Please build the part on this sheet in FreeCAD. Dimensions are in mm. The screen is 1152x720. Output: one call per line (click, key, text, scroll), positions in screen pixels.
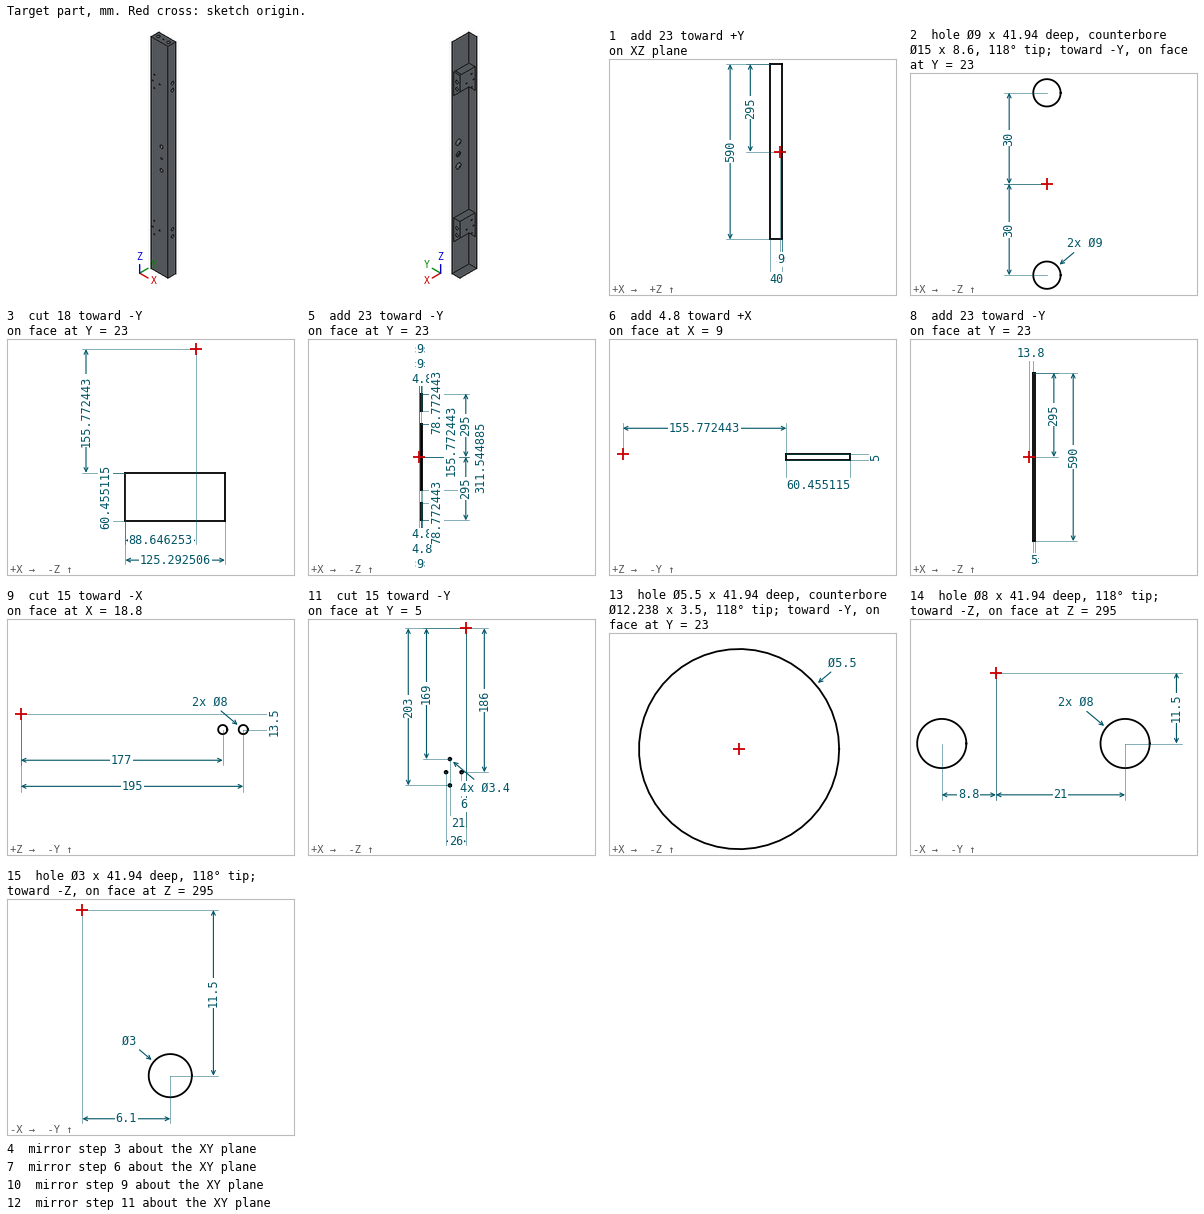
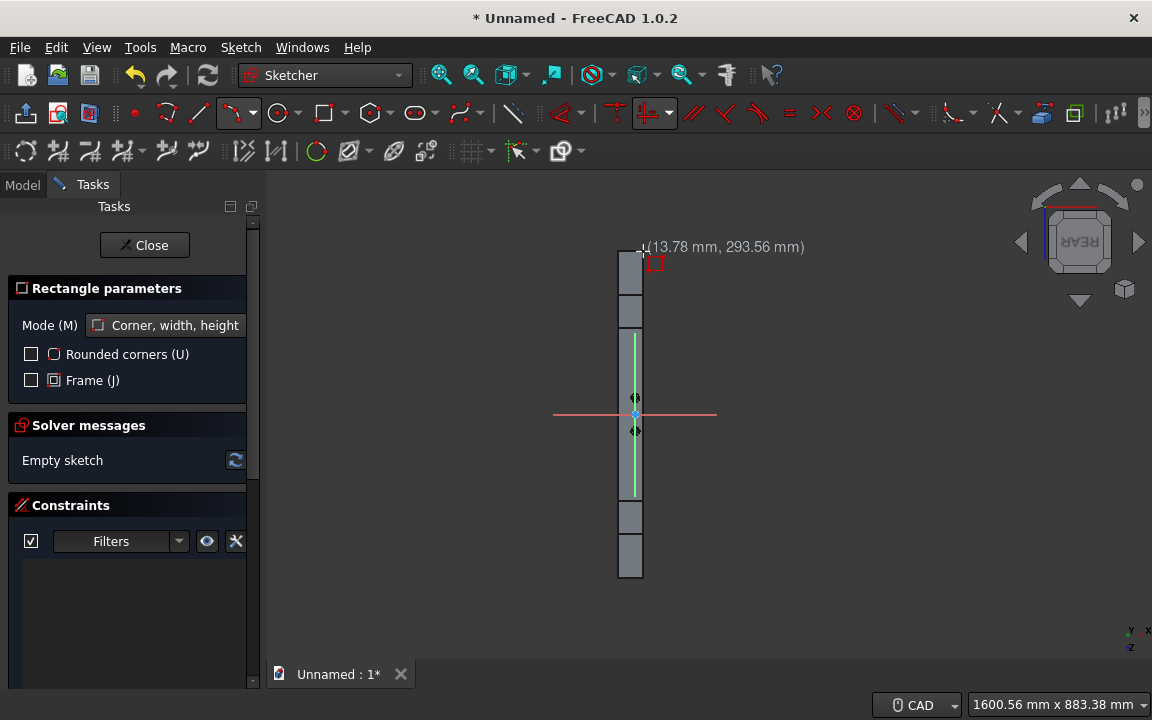
scroll(643, 251, up, 4)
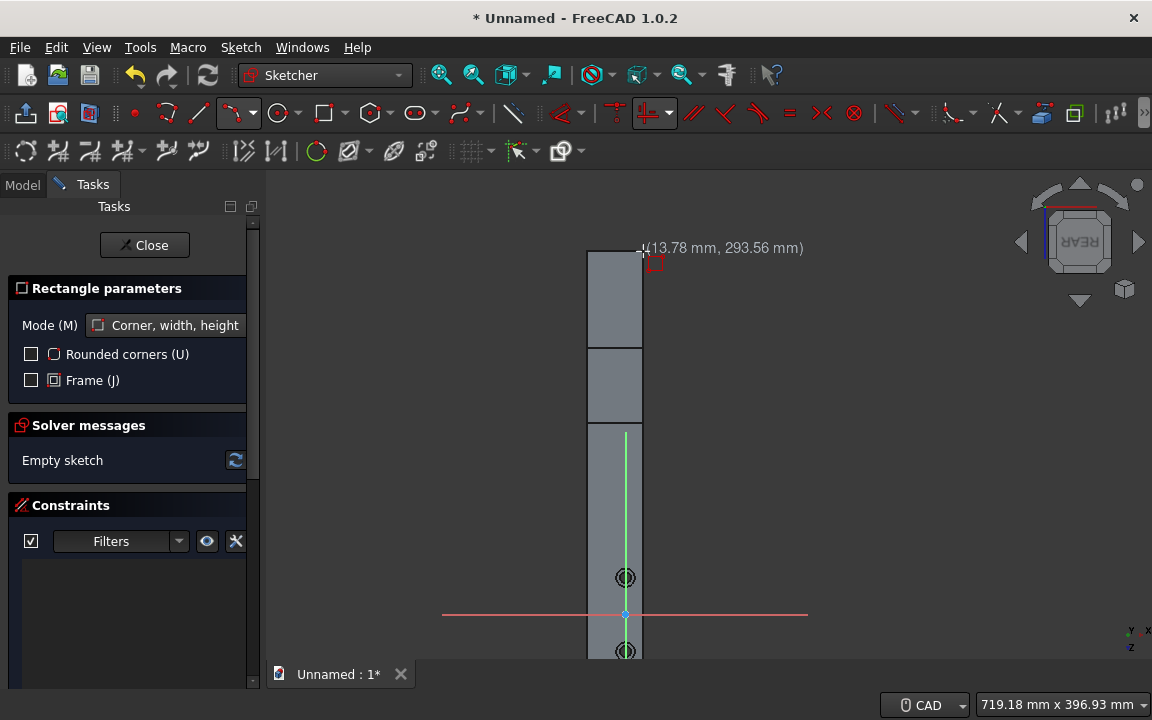
click(643, 251)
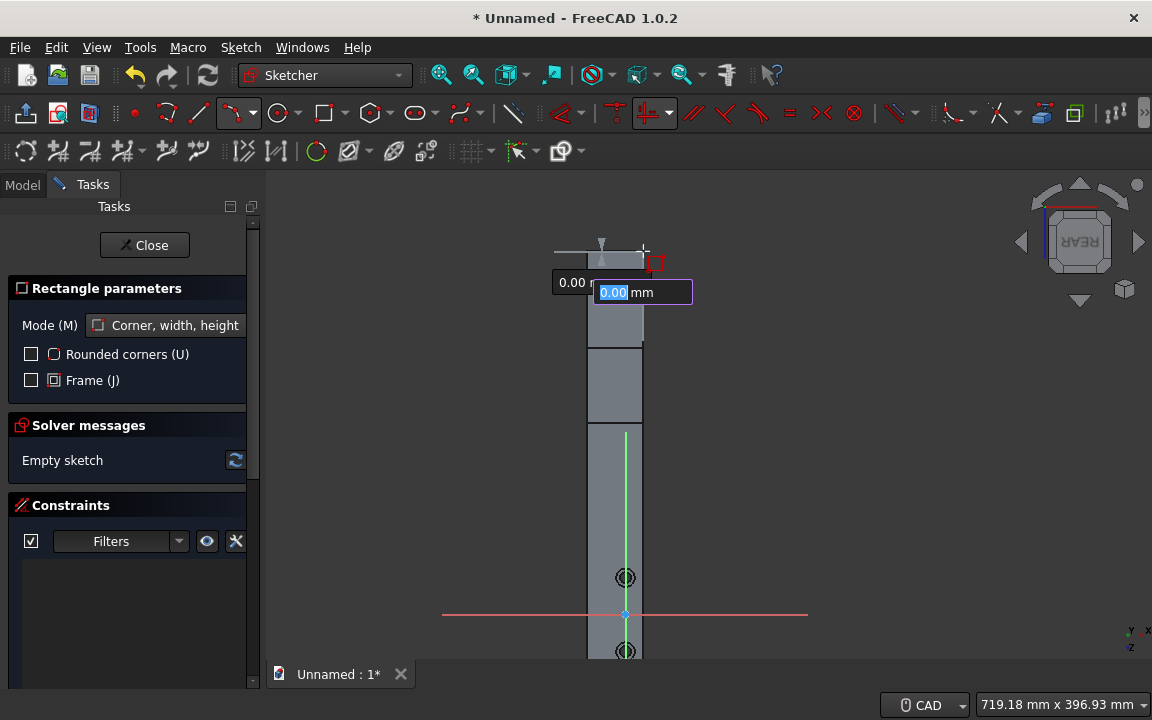
scroll(643, 251, down, 4)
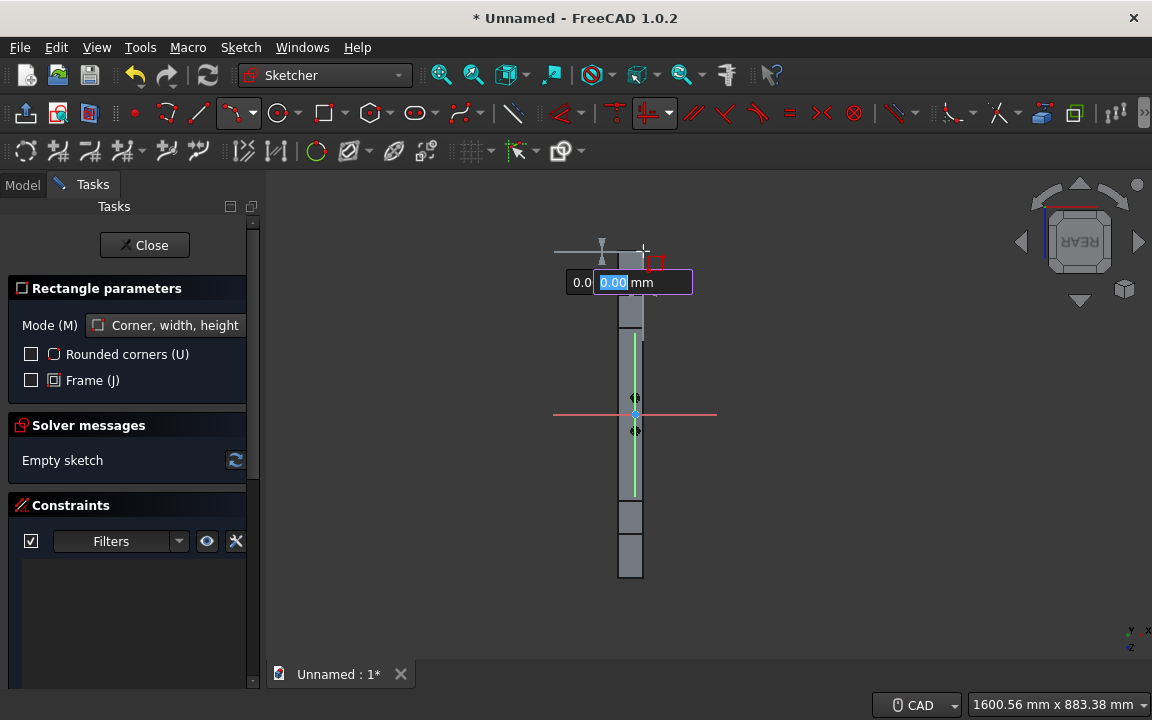
scroll(646, 578, up, 3)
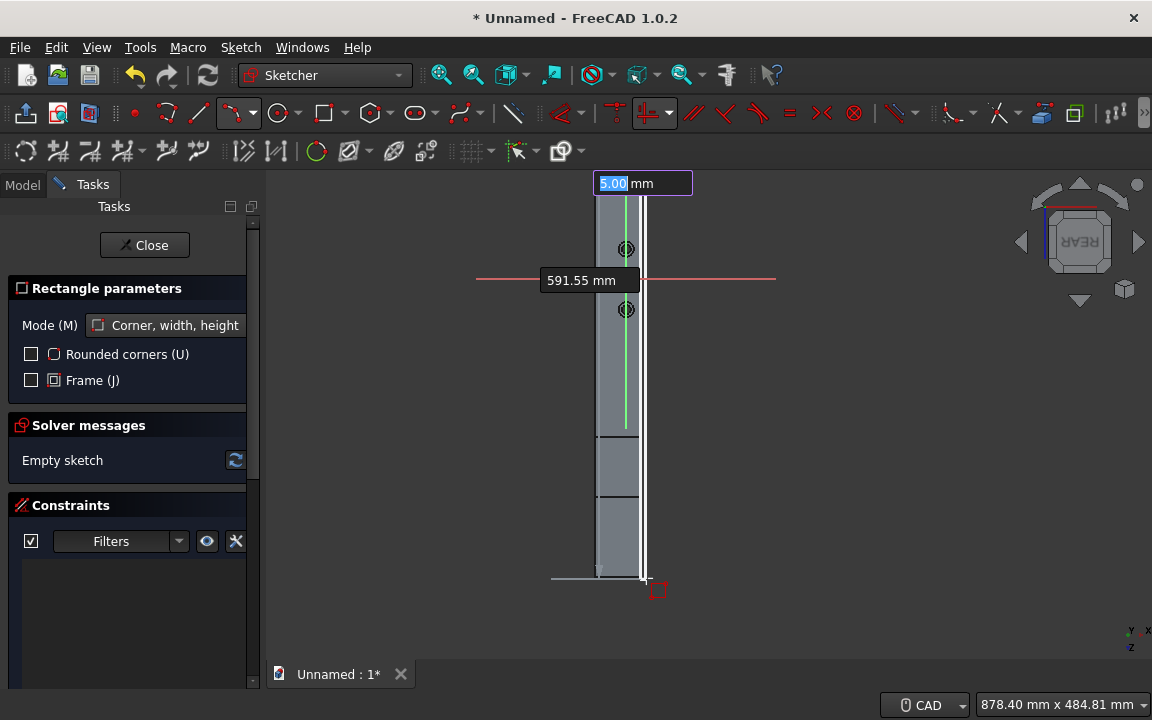
click(645, 577)
key(Escape)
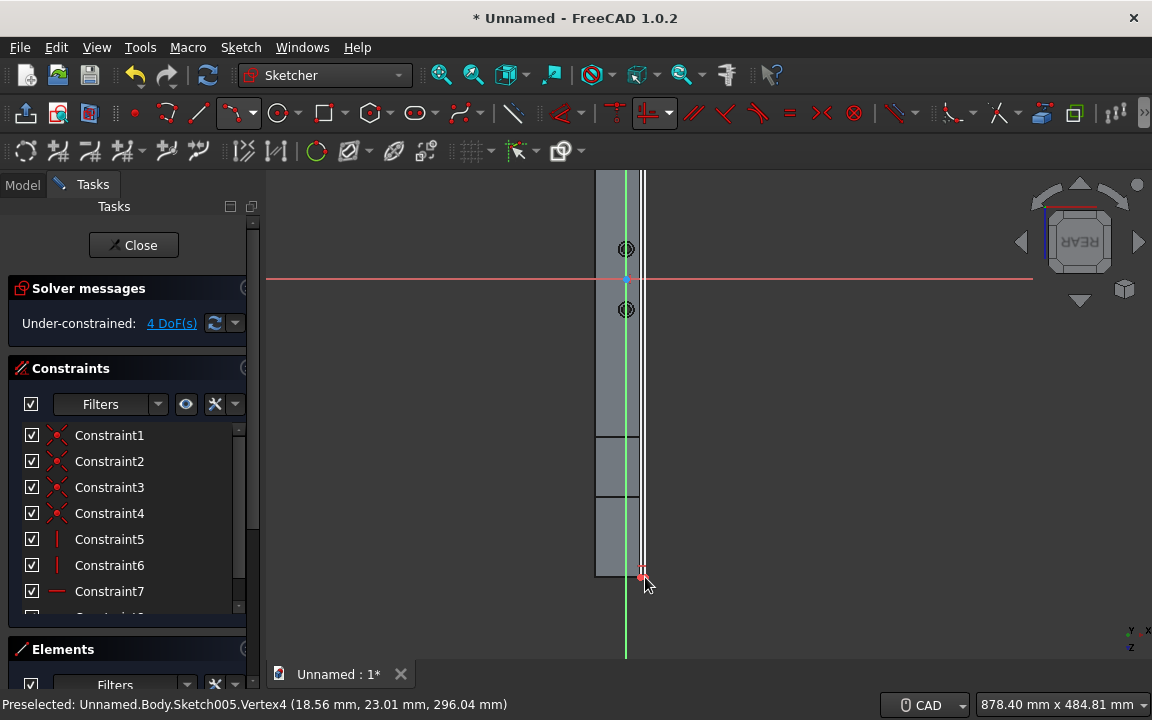
click(560, 114)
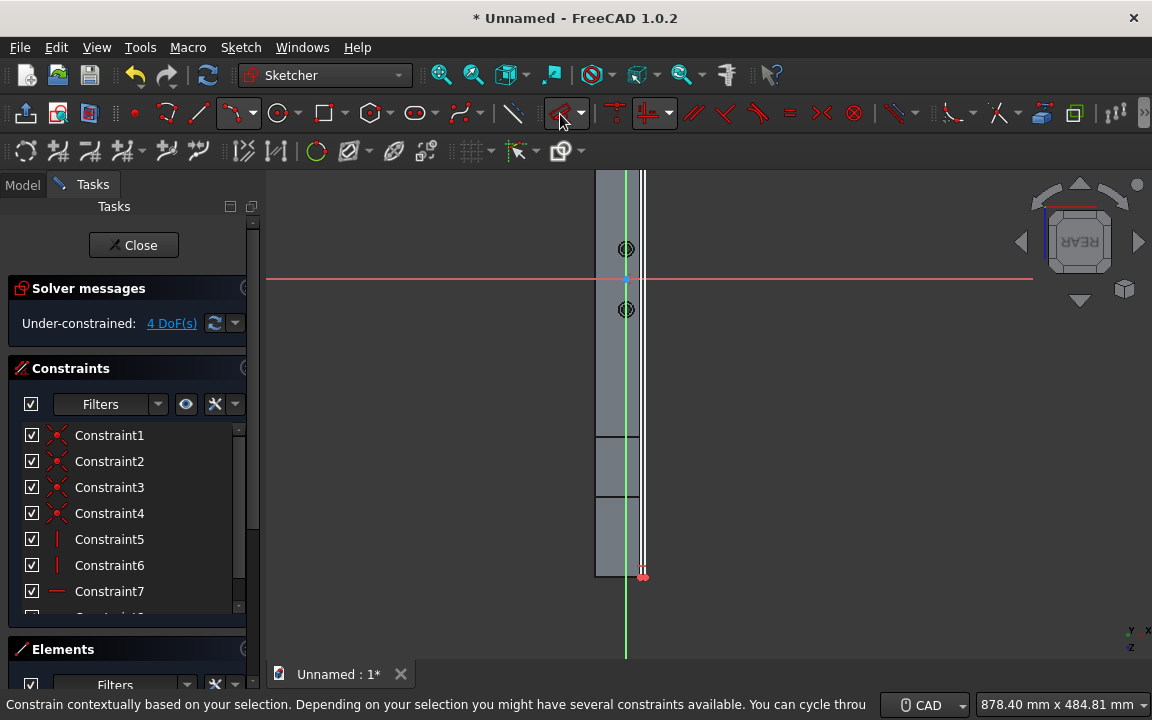
scroll(643, 578, up, 11)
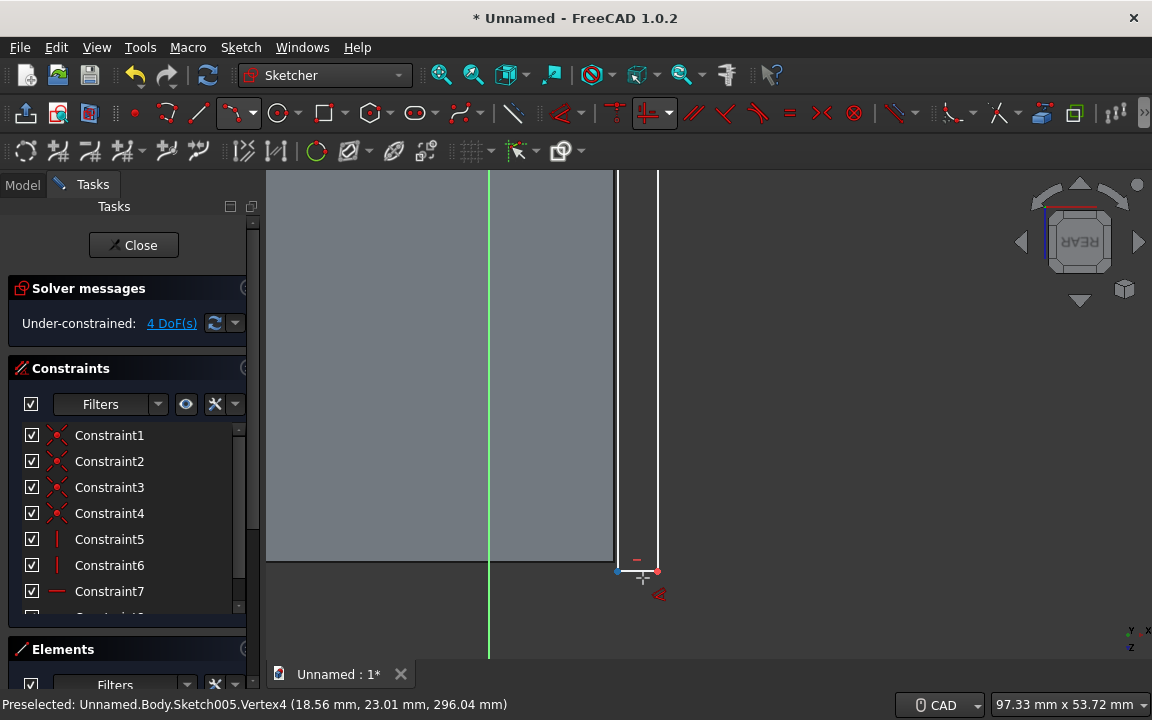
click(638, 571)
click(638, 605)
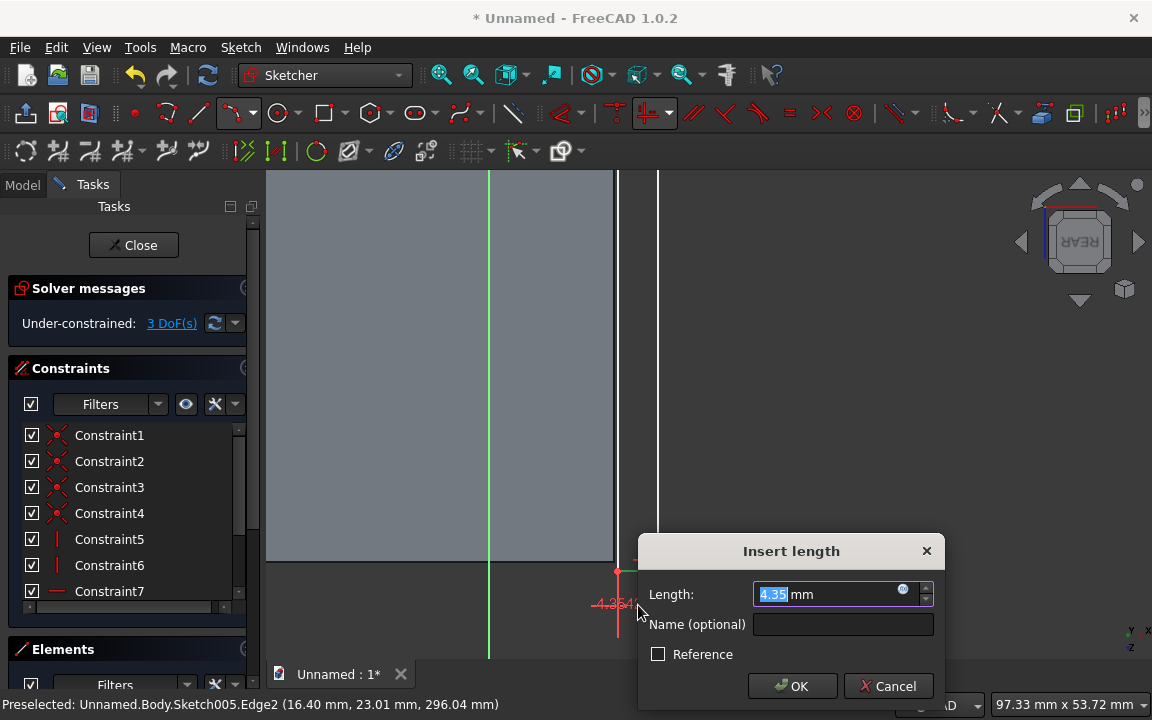
text(5)
key(Return)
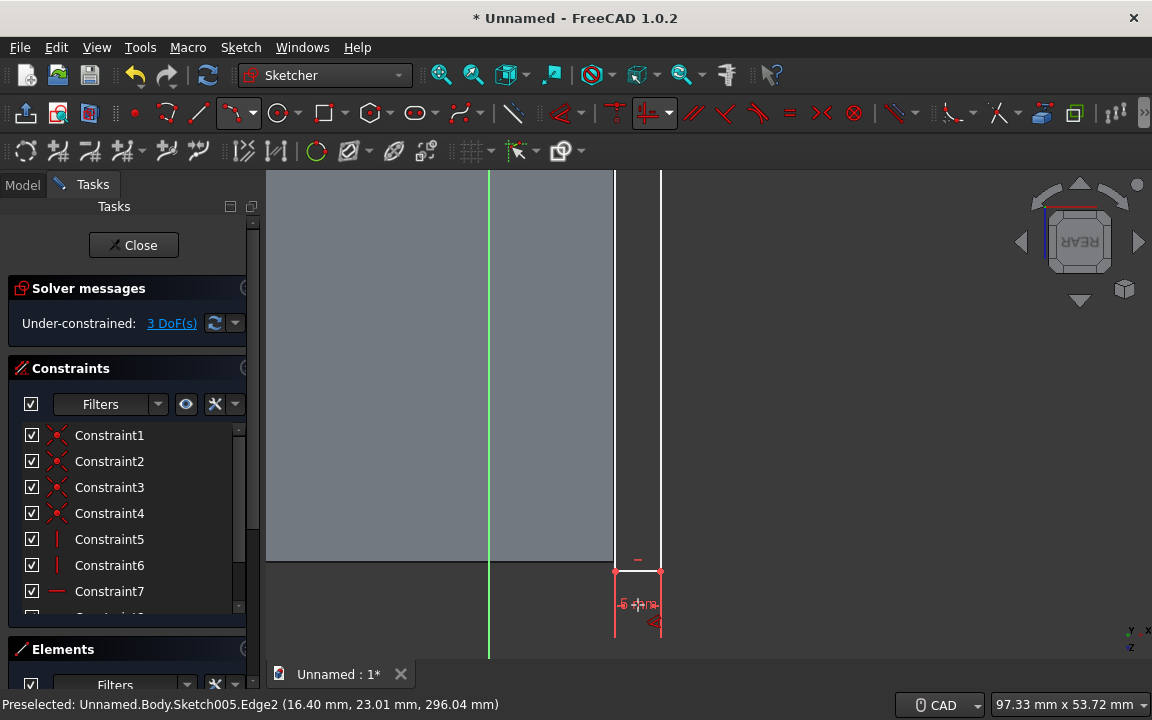
scroll(645, 579, down, 14)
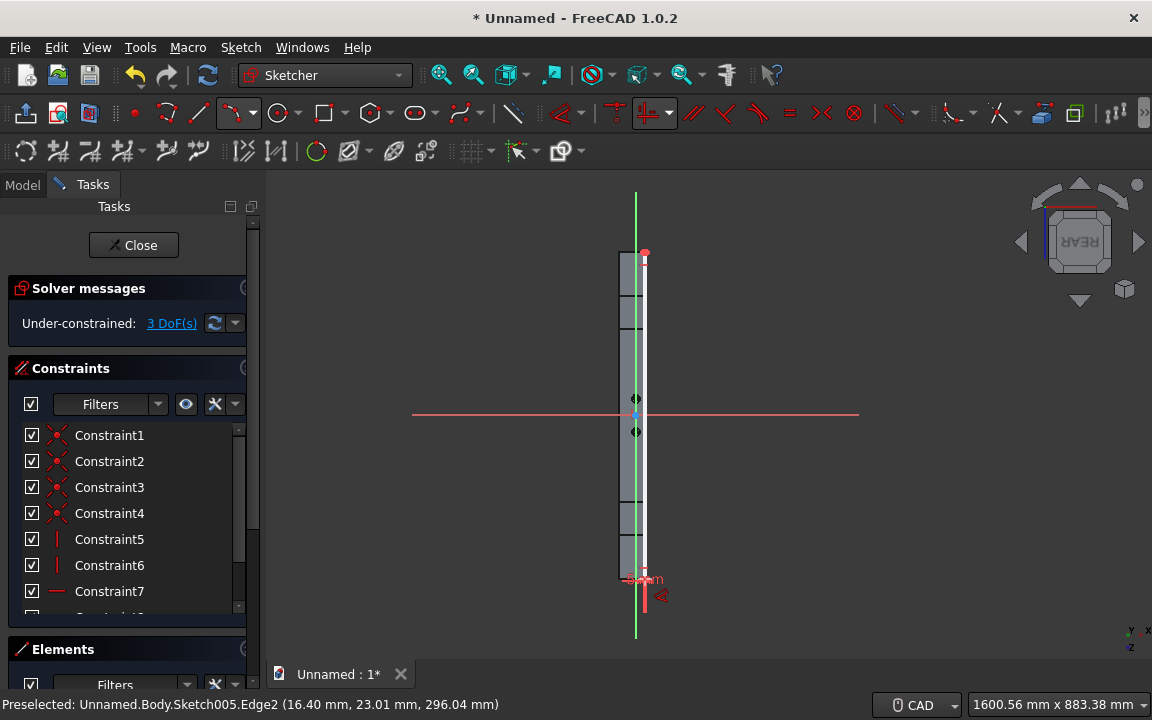
scroll(644, 351, up, 9)